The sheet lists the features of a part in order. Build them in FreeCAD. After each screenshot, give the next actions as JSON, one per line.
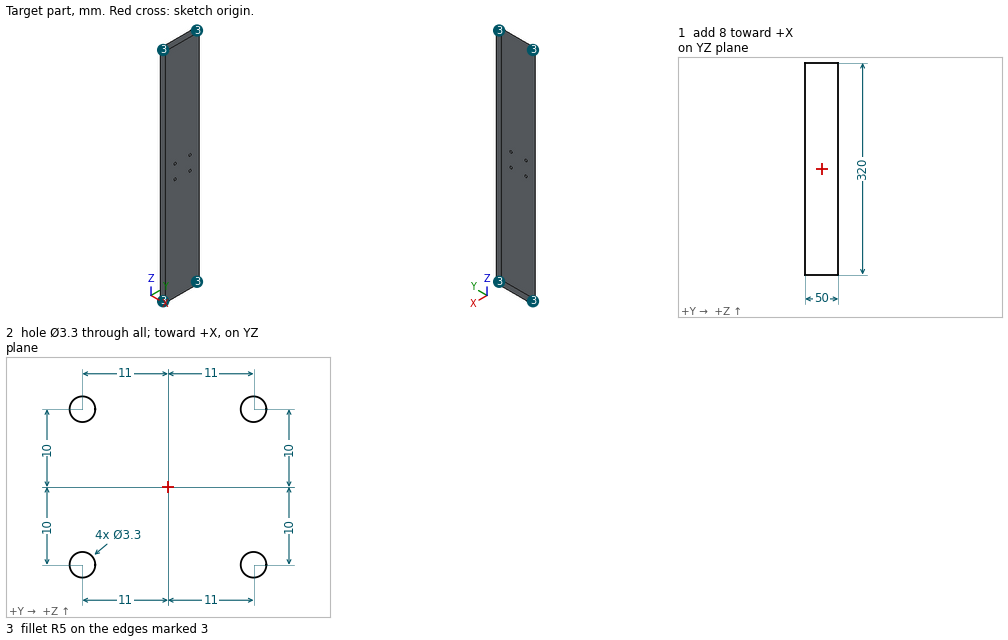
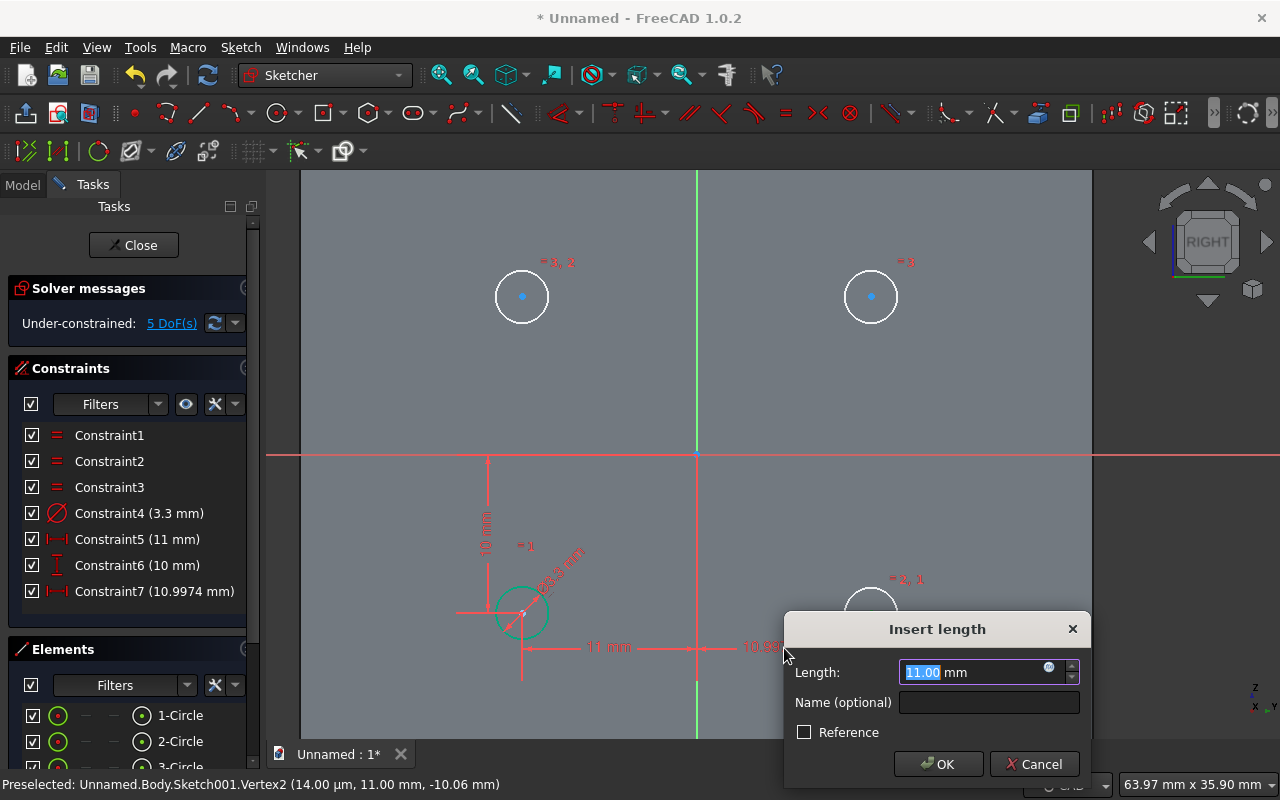
{"action": "type", "text": "11"}
{"action": "key", "text": "Return"}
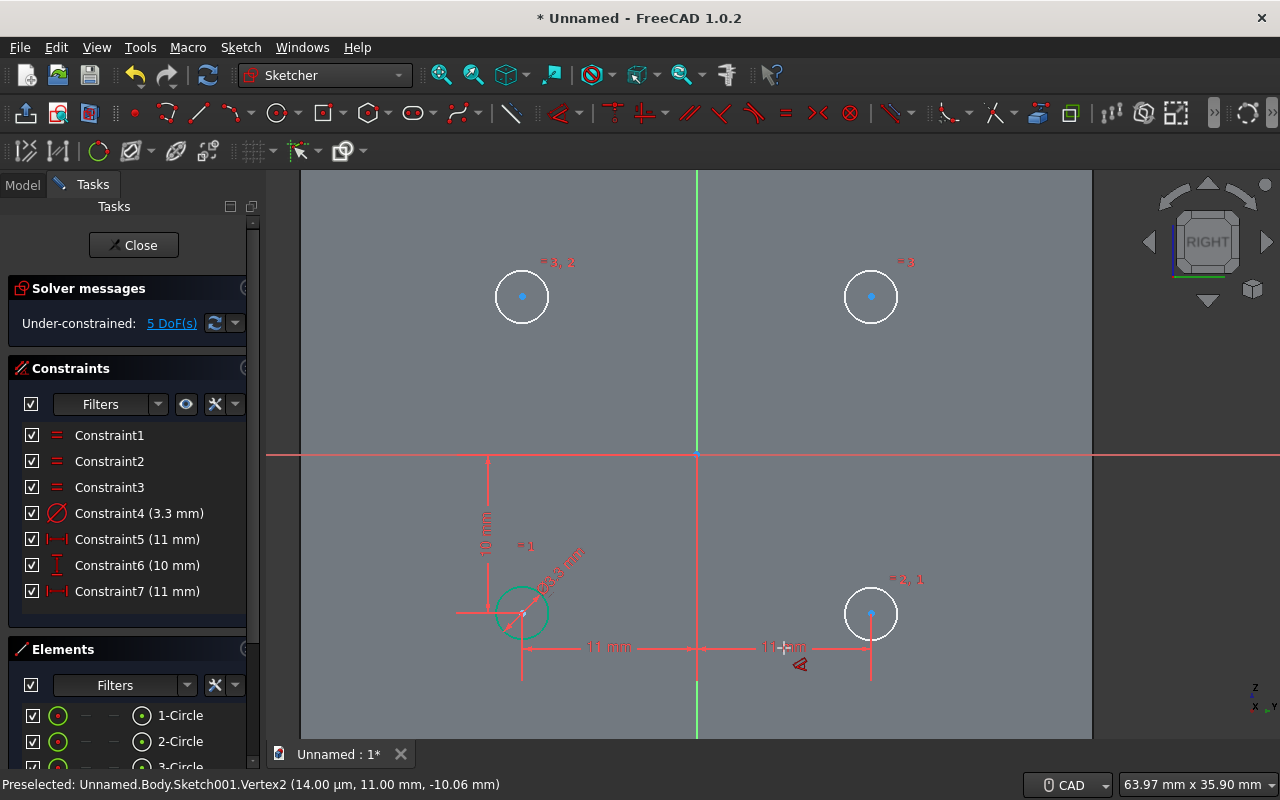
{"action": "left_click", "coordinate": [871, 614]}
{"action": "left_click", "coordinate": [905, 534]}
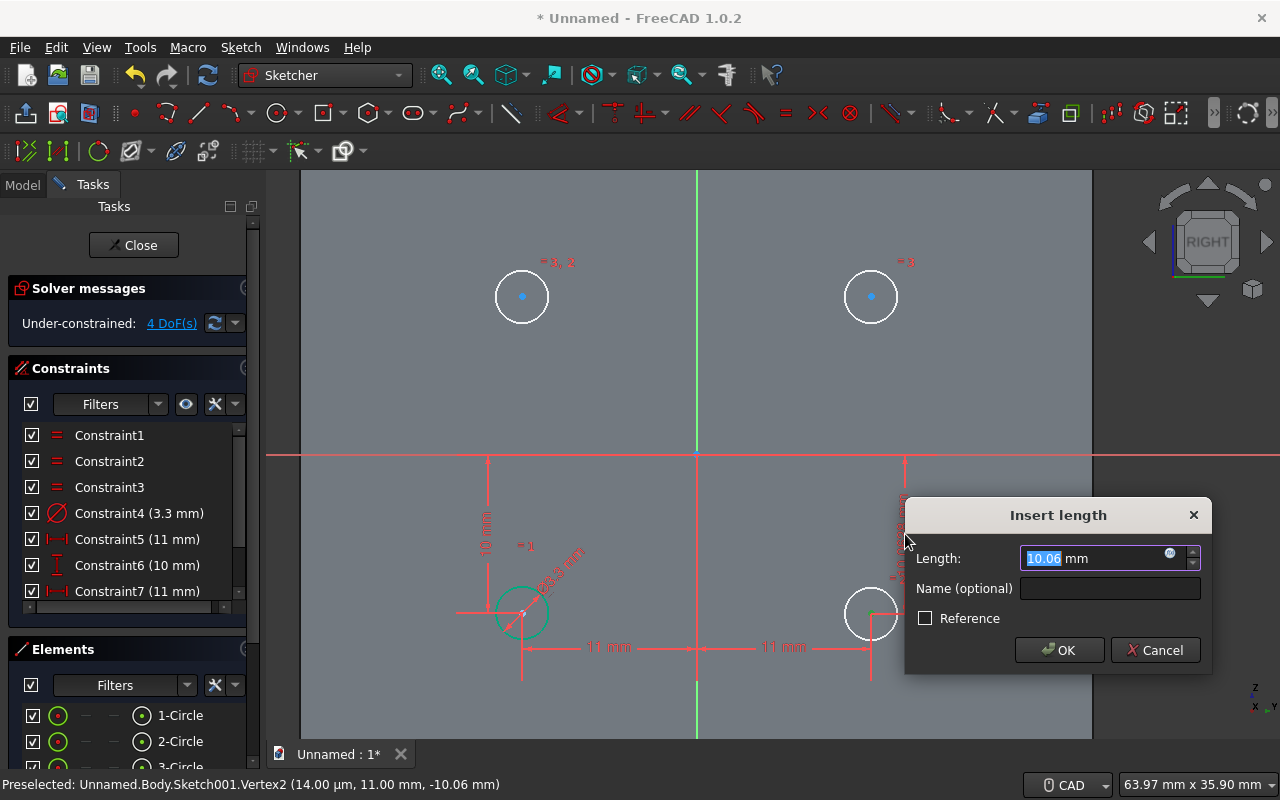
{"action": "type", "text": "10"}
{"action": "key", "text": "Return"}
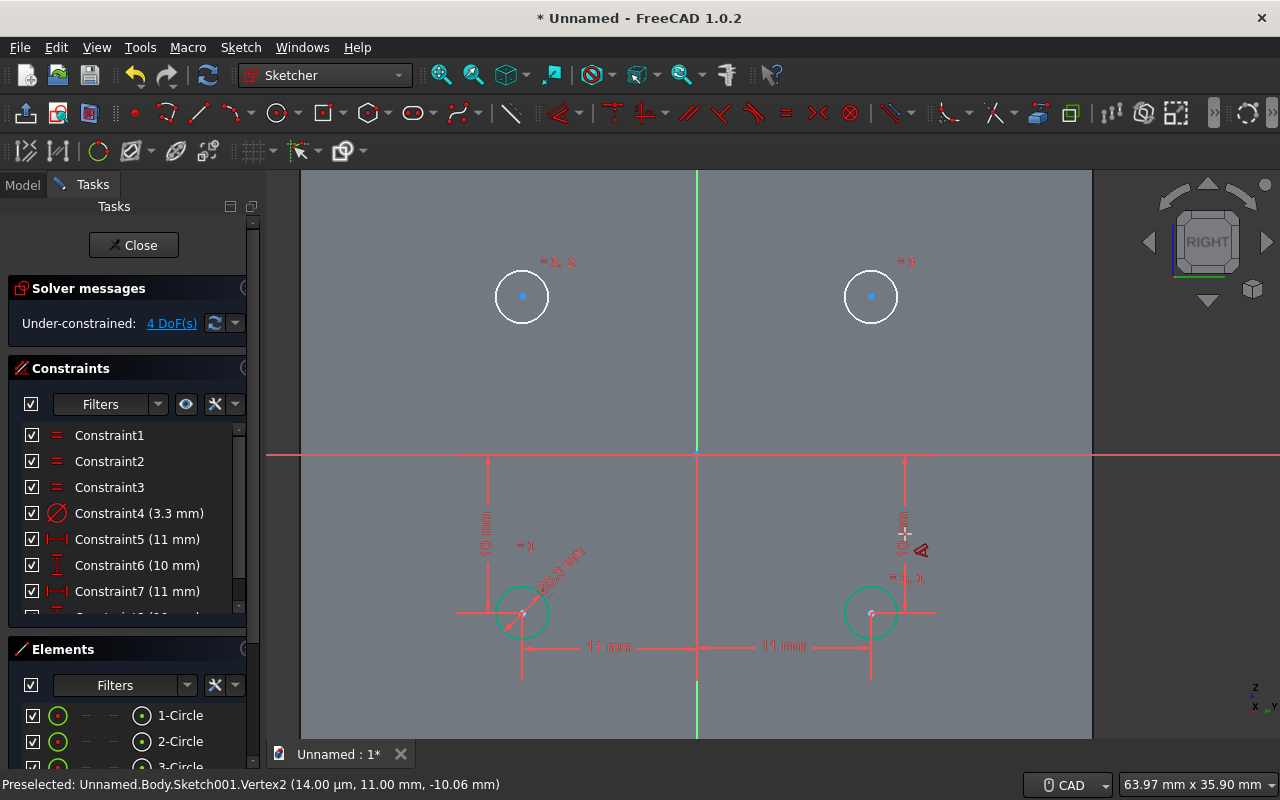
{"action": "left_click", "coordinate": [522, 297]}
{"action": "left_click", "coordinate": [609, 263]}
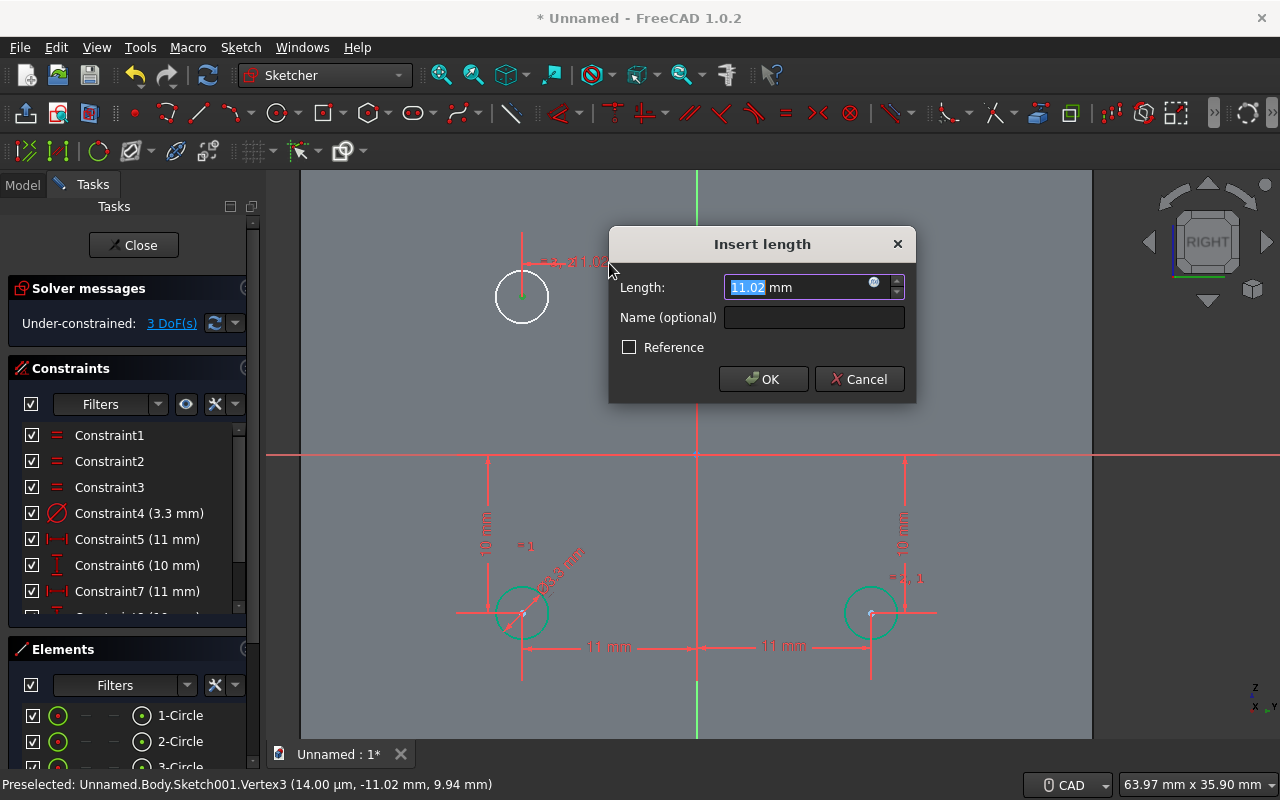
{"action": "type", "text": "11"}
{"action": "key", "text": "Return"}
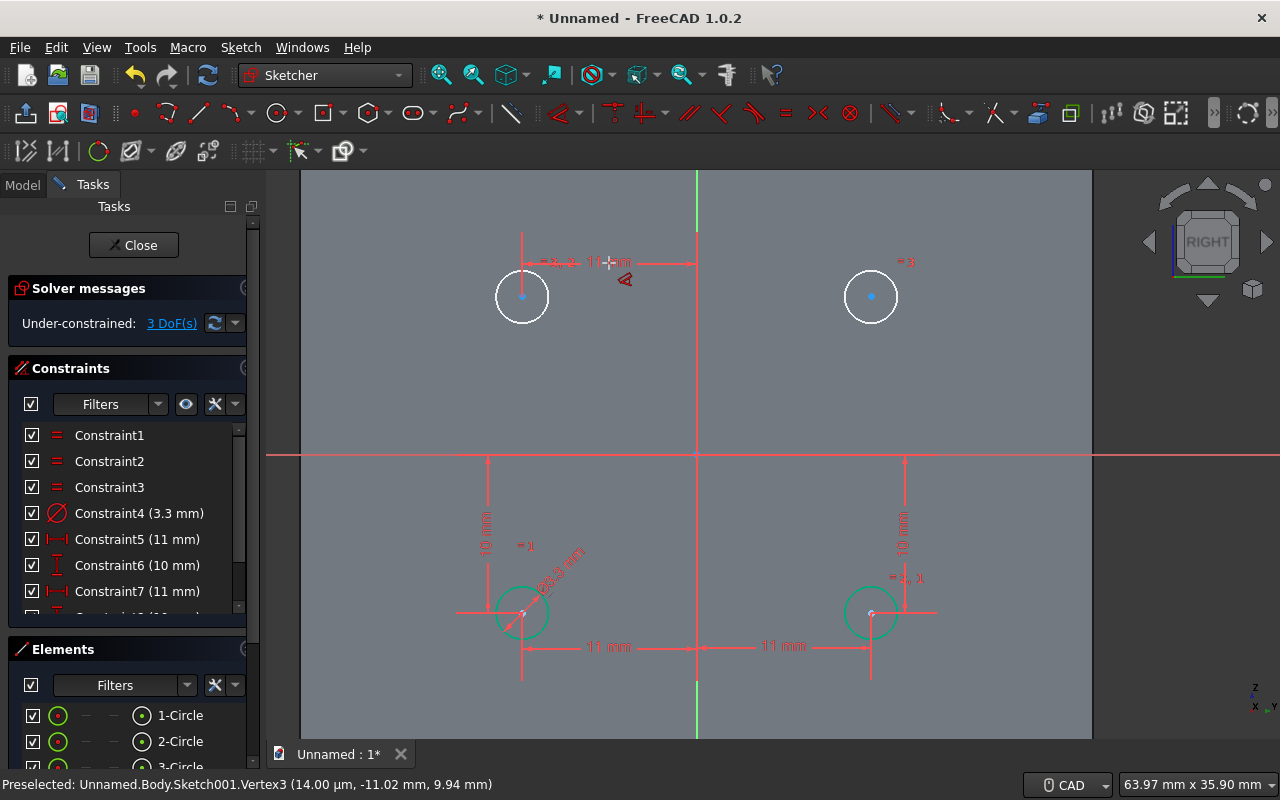
{"action": "left_click", "coordinate": [522, 297]}
{"action": "left_click", "coordinate": [488, 376]}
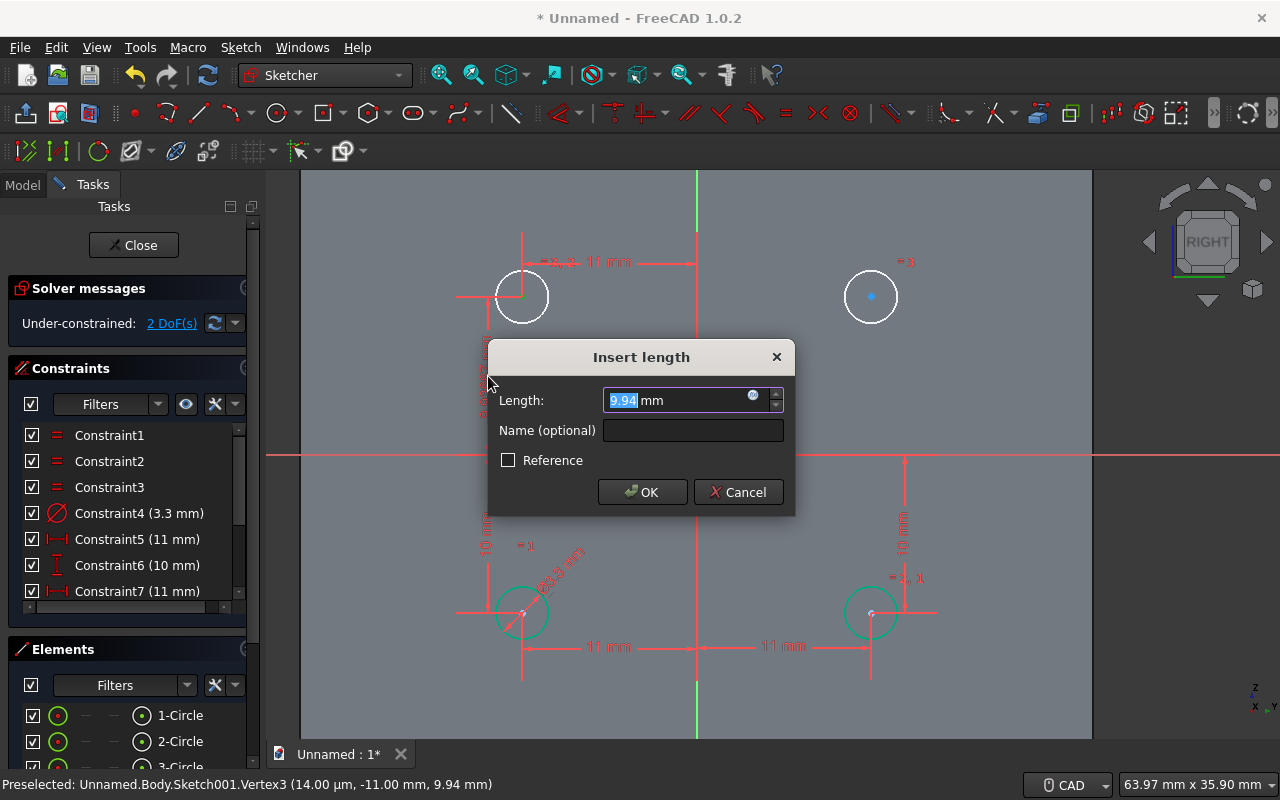
{"action": "type", "text": "10"}
{"action": "key", "text": "Return"}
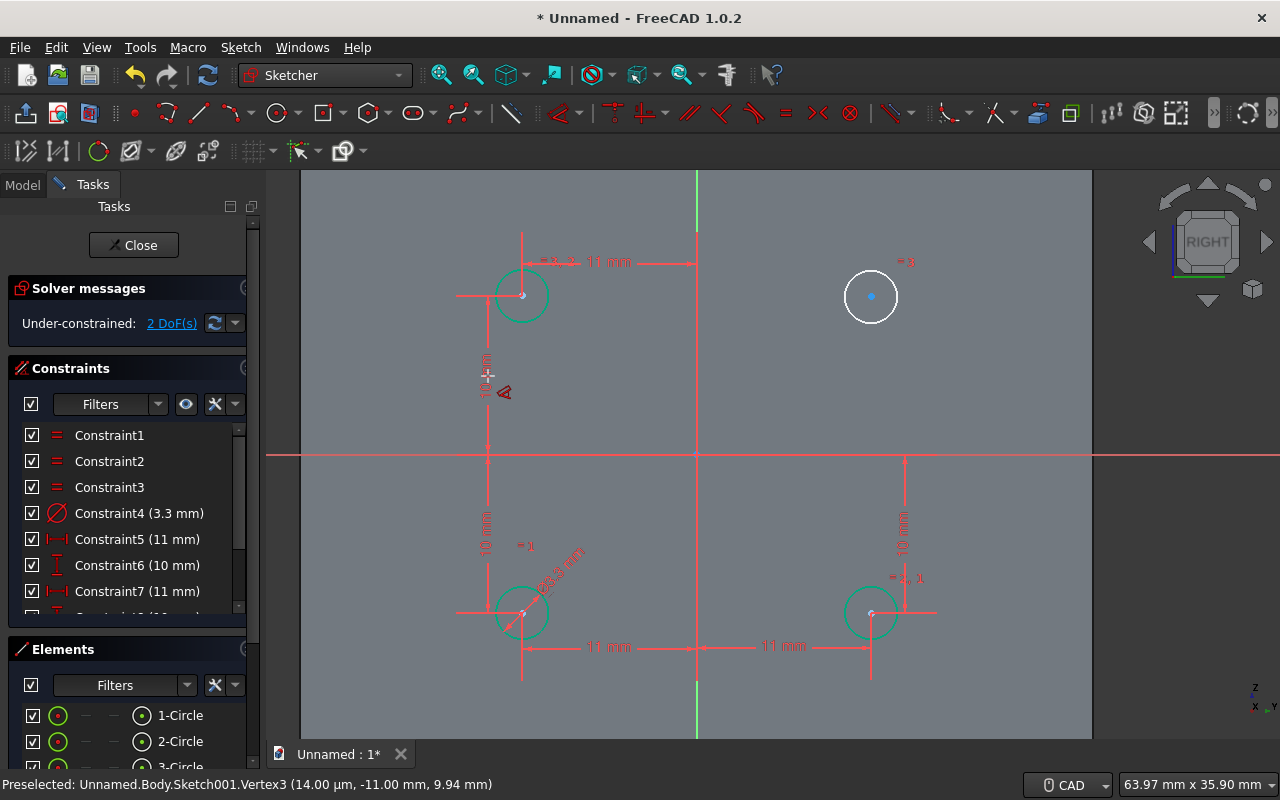
{"action": "left_click", "coordinate": [871, 297]}
{"action": "left_click", "coordinate": [784, 263]}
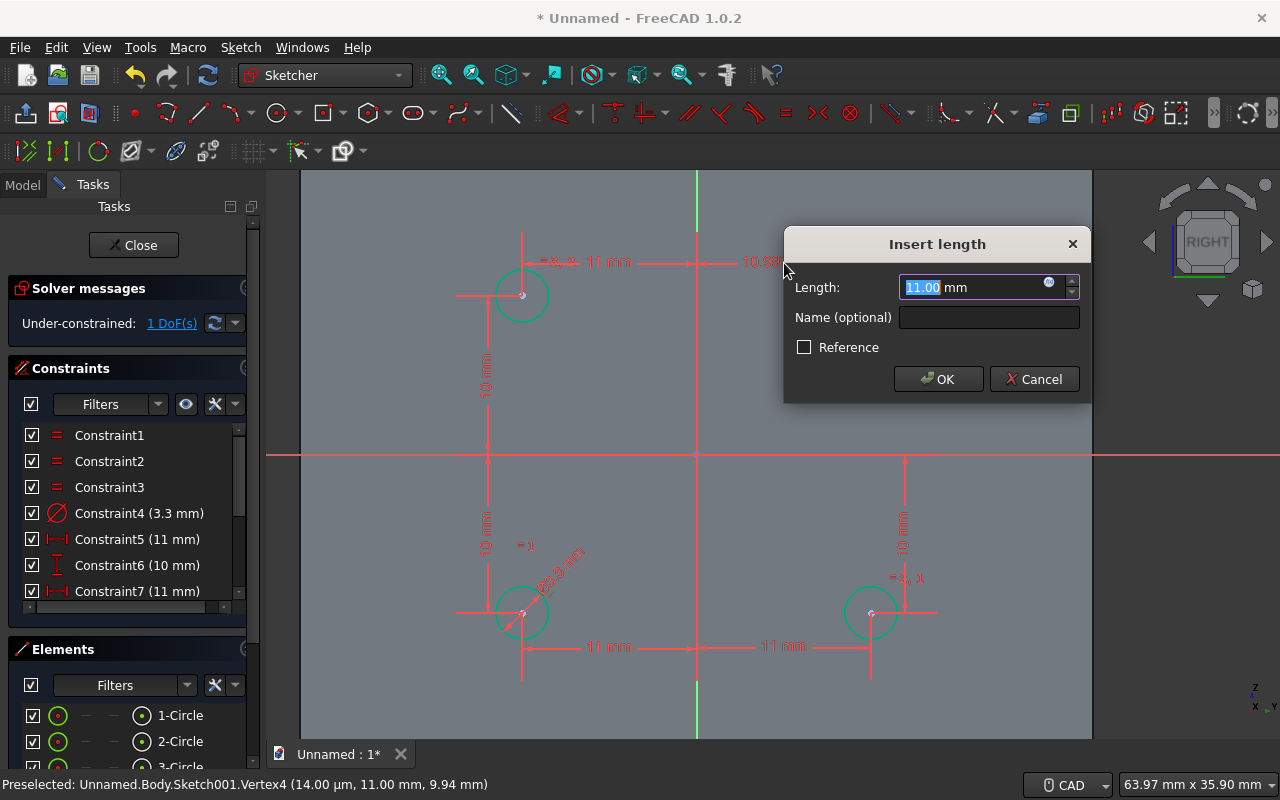
{"action": "type", "text": "11"}
{"action": "key", "text": "Return"}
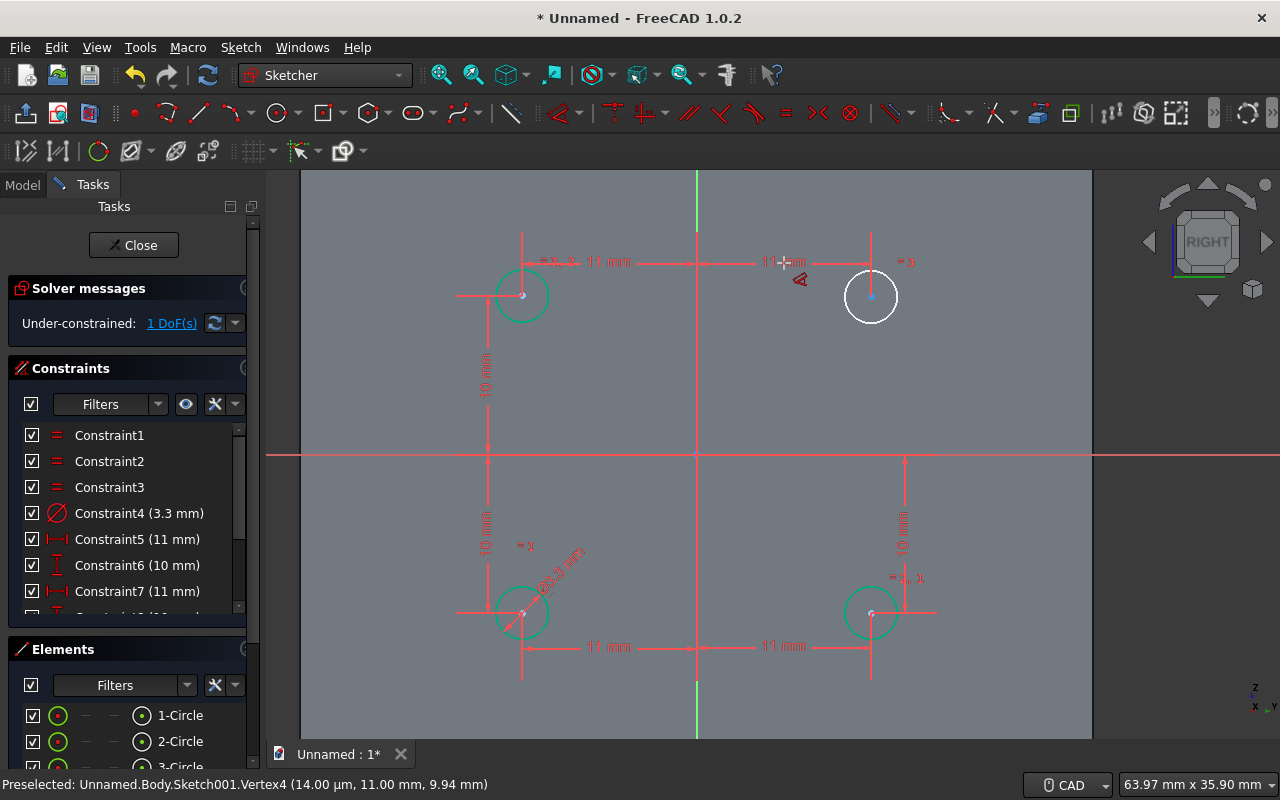
{"action": "left_click", "coordinate": [871, 297]}
{"action": "left_click", "coordinate": [905, 376]}